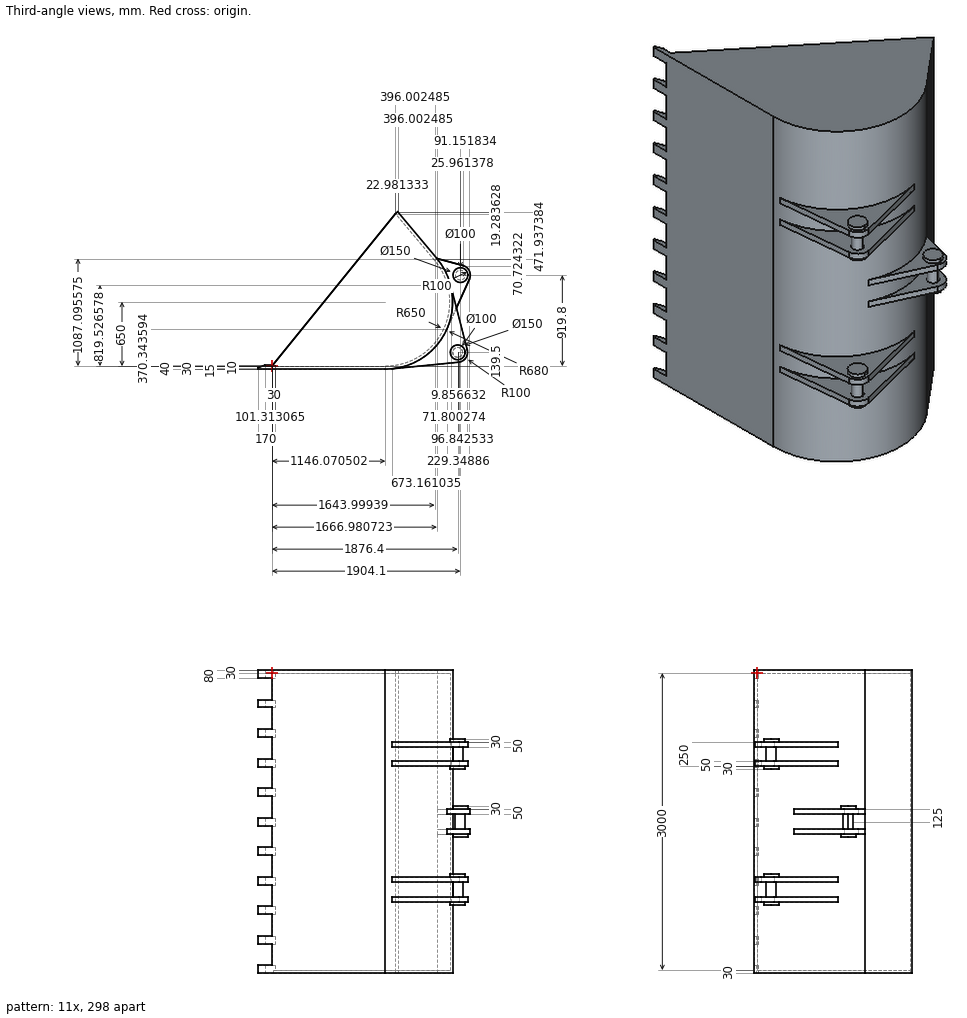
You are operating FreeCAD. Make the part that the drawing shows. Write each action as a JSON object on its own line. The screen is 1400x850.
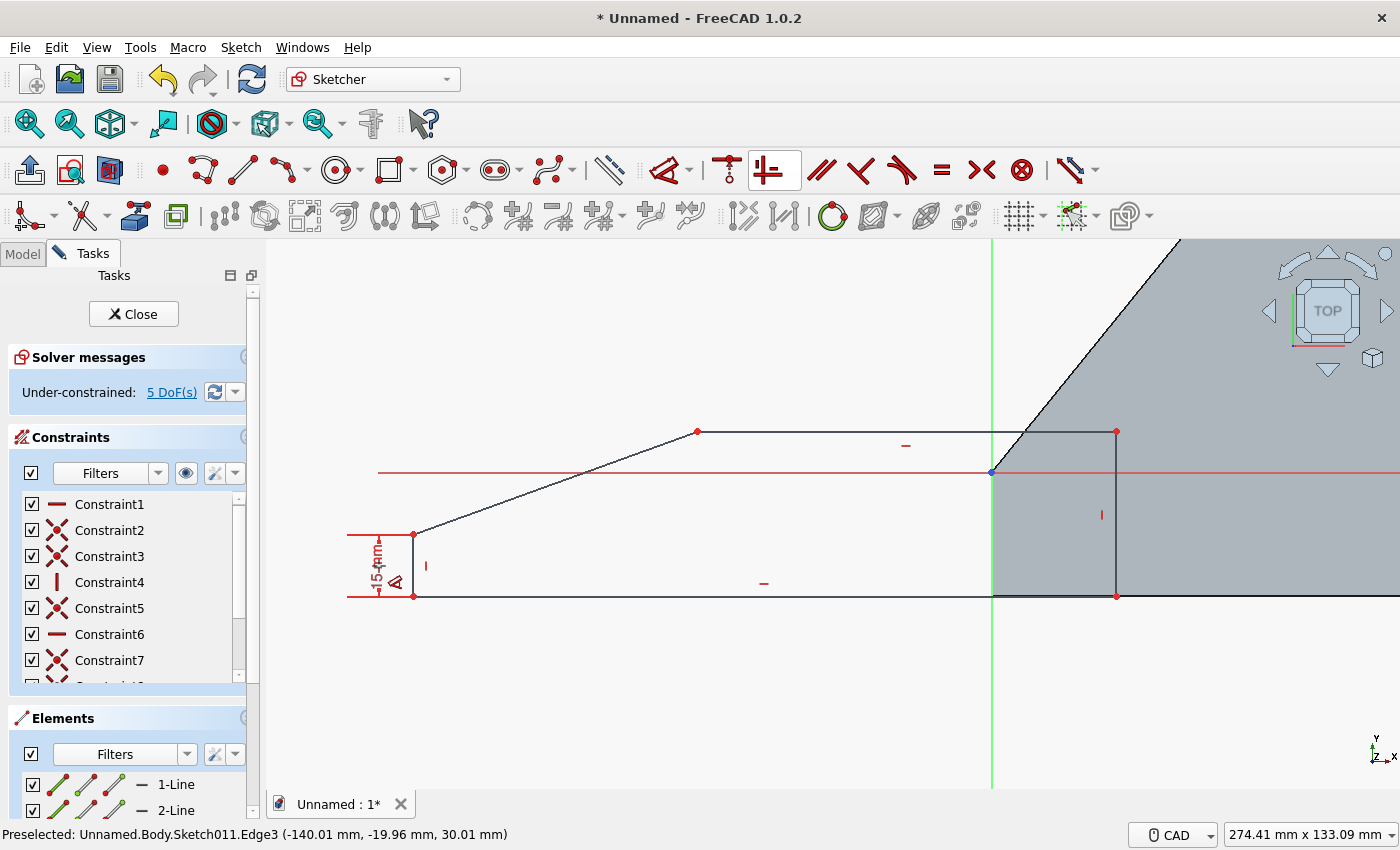
{"action": "left_click", "coordinate": [1116, 547]}
{"action": "left_click", "coordinate": [1150, 514]}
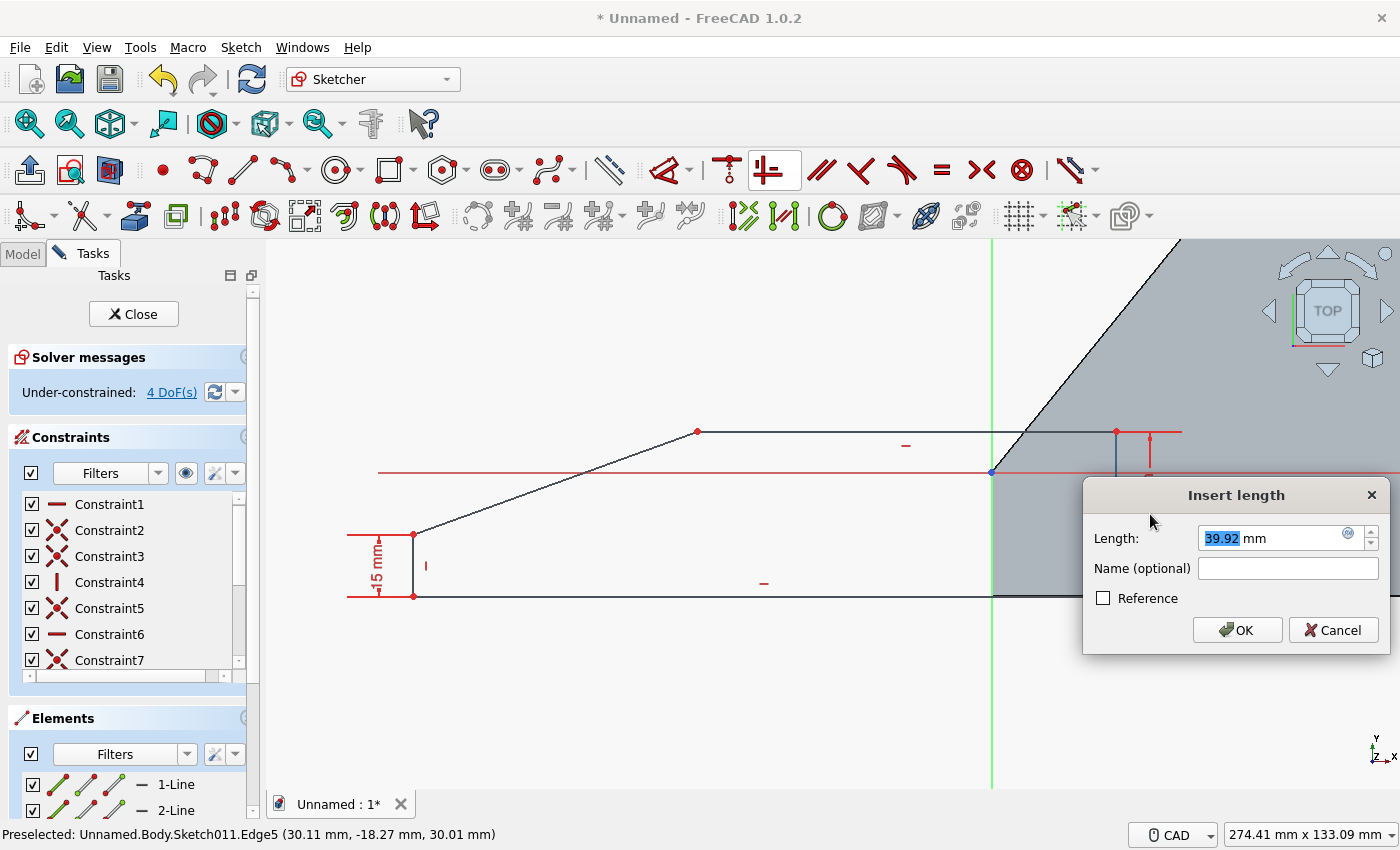
{"action": "type", "text": "40"}
{"action": "key", "text": "Return"}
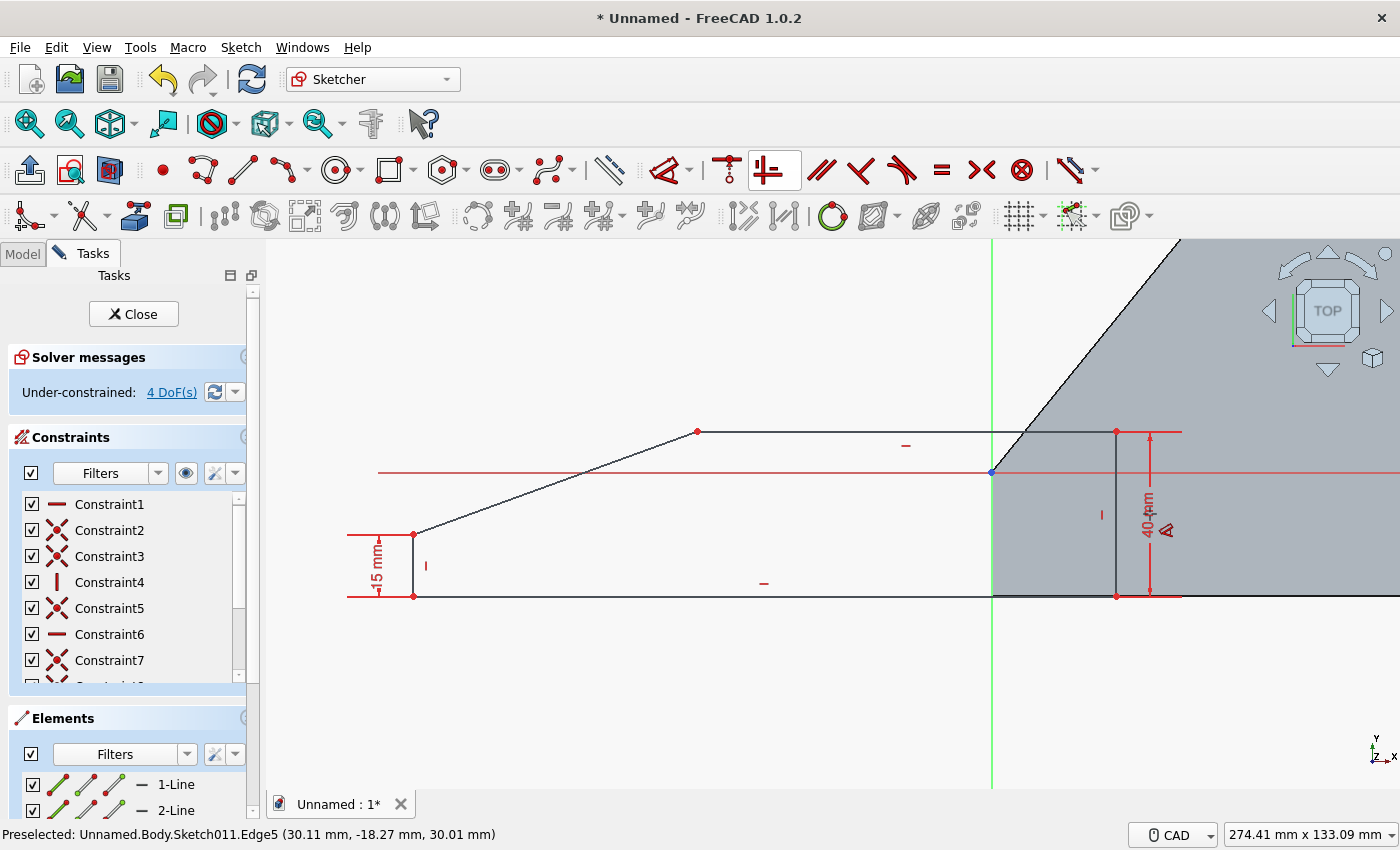
{"action": "left_click", "coordinate": [624, 597]}
{"action": "left_click", "coordinate": [764, 631]}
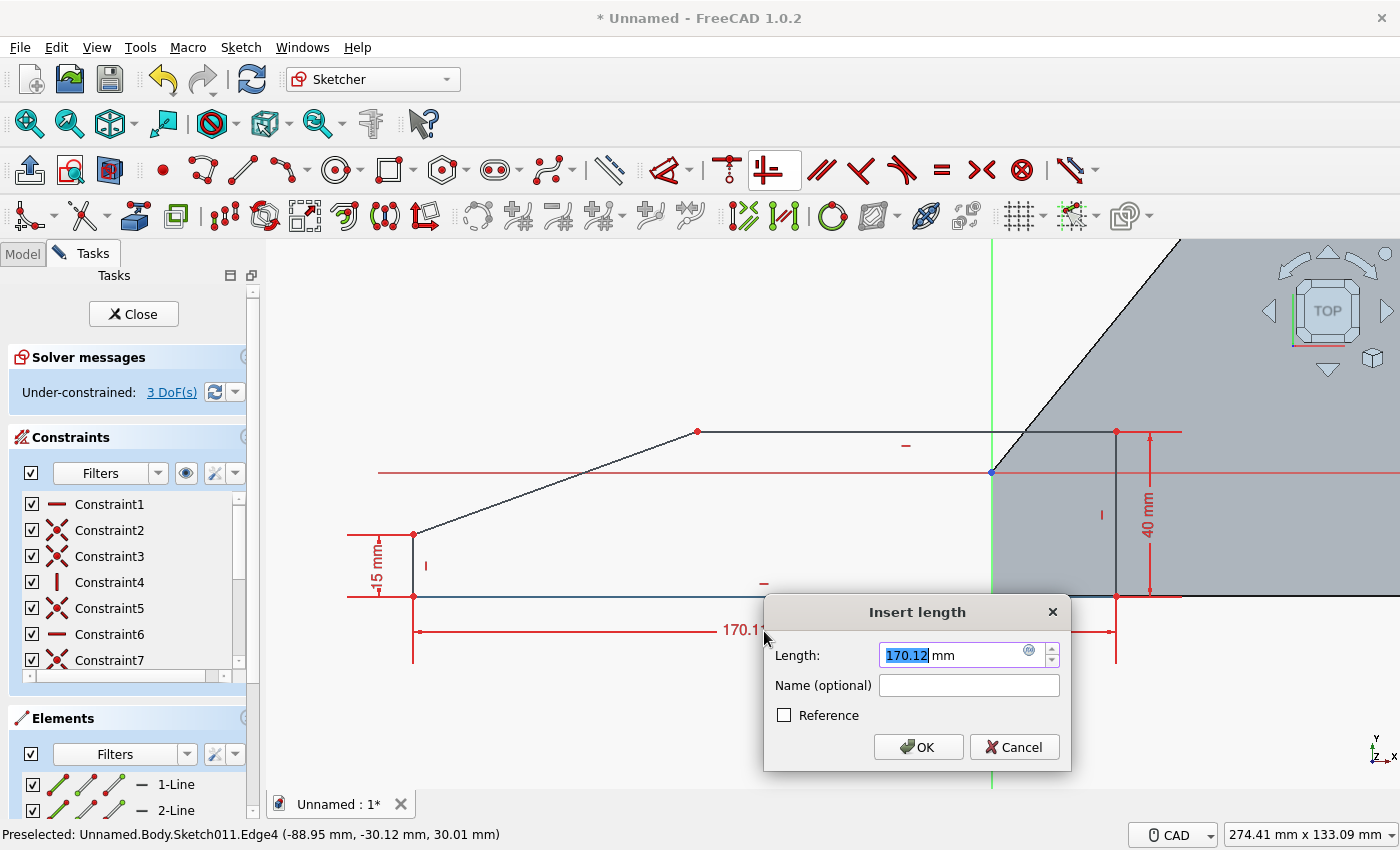
{"action": "type", "text": "170"}
{"action": "key", "text": "Return"}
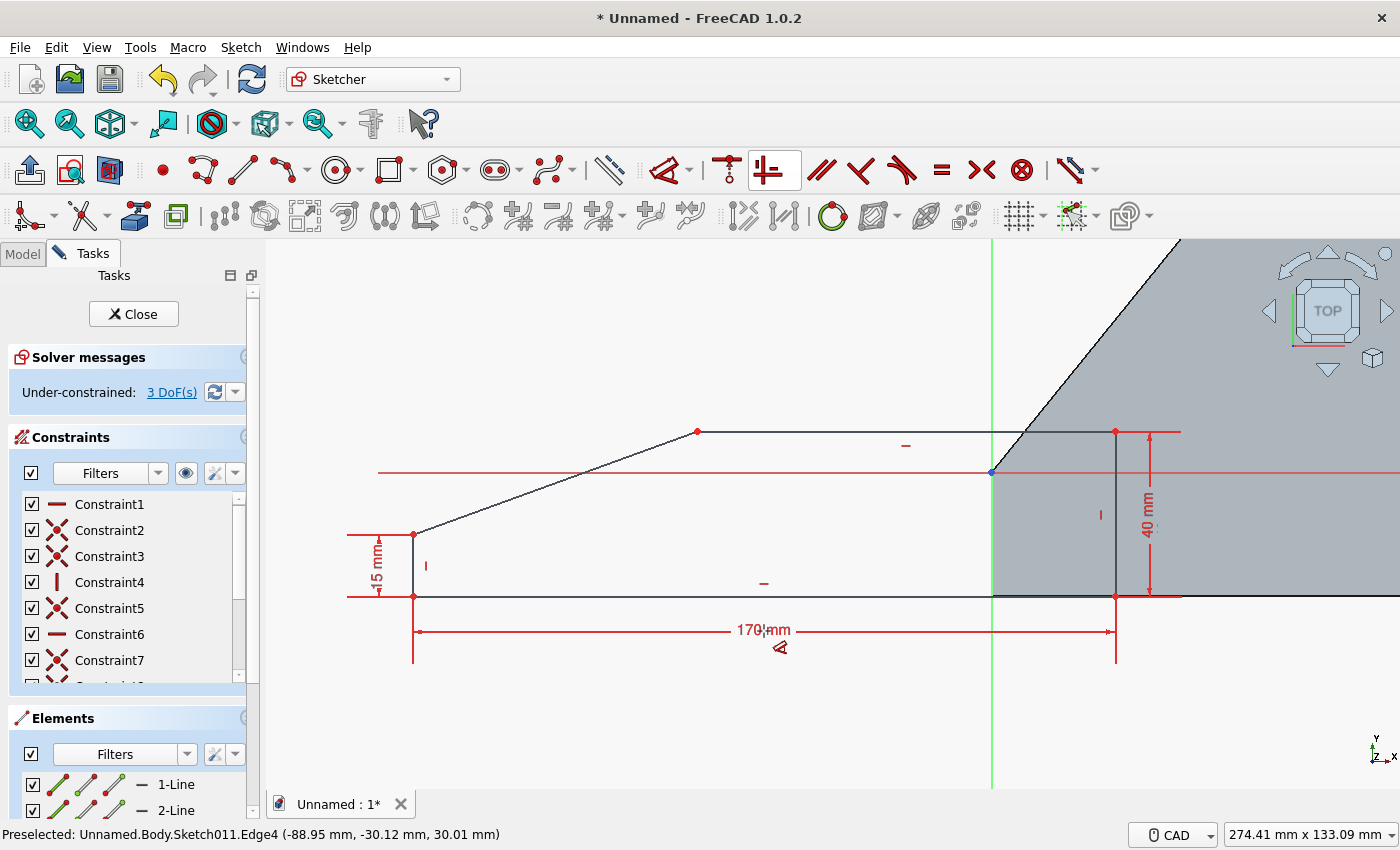
{"action": "left_click", "coordinate": [1116, 432]}
{"action": "left_click", "coordinate": [1054, 398]}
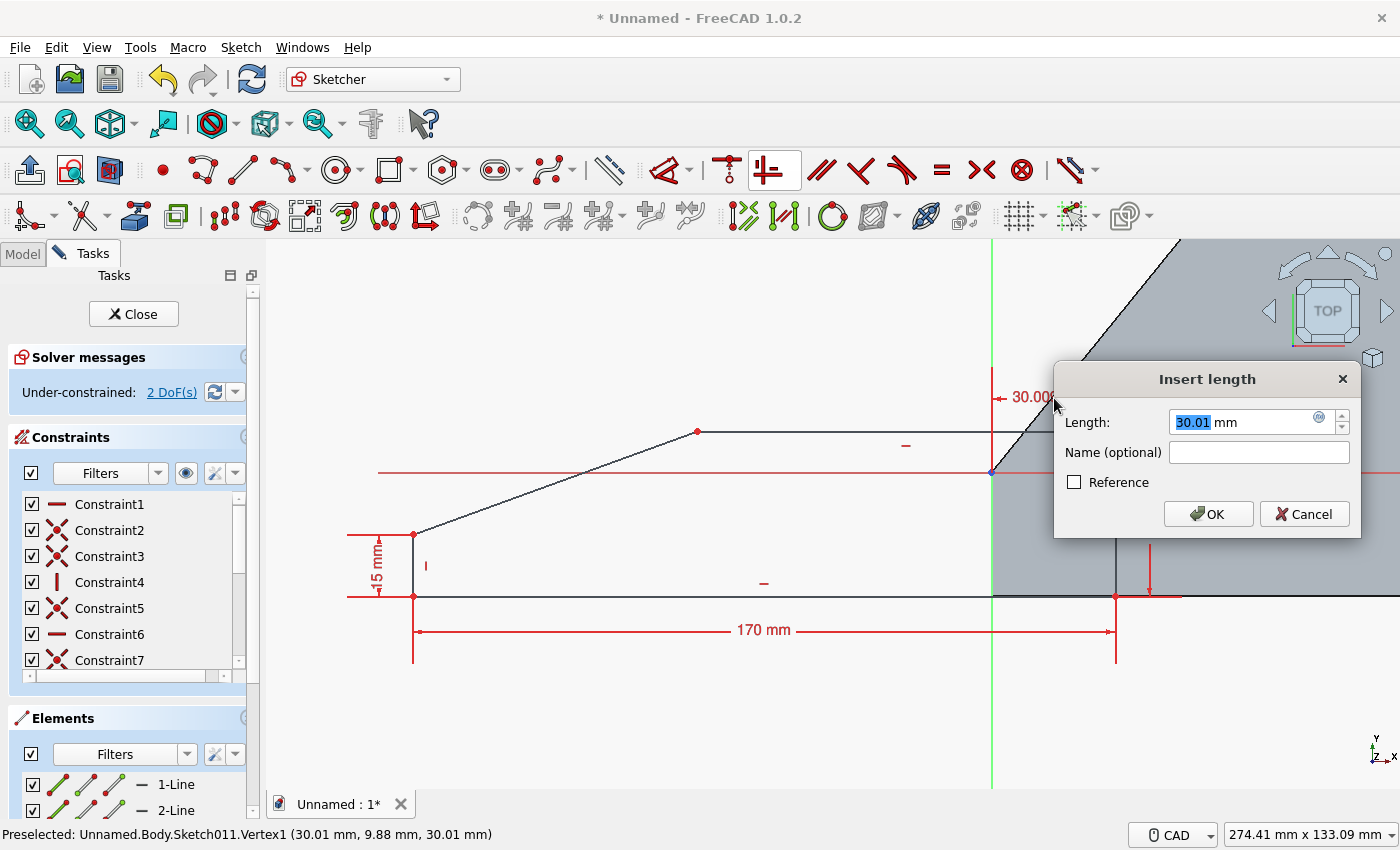
{"action": "type", "text": "30"}
{"action": "key", "text": "Return"}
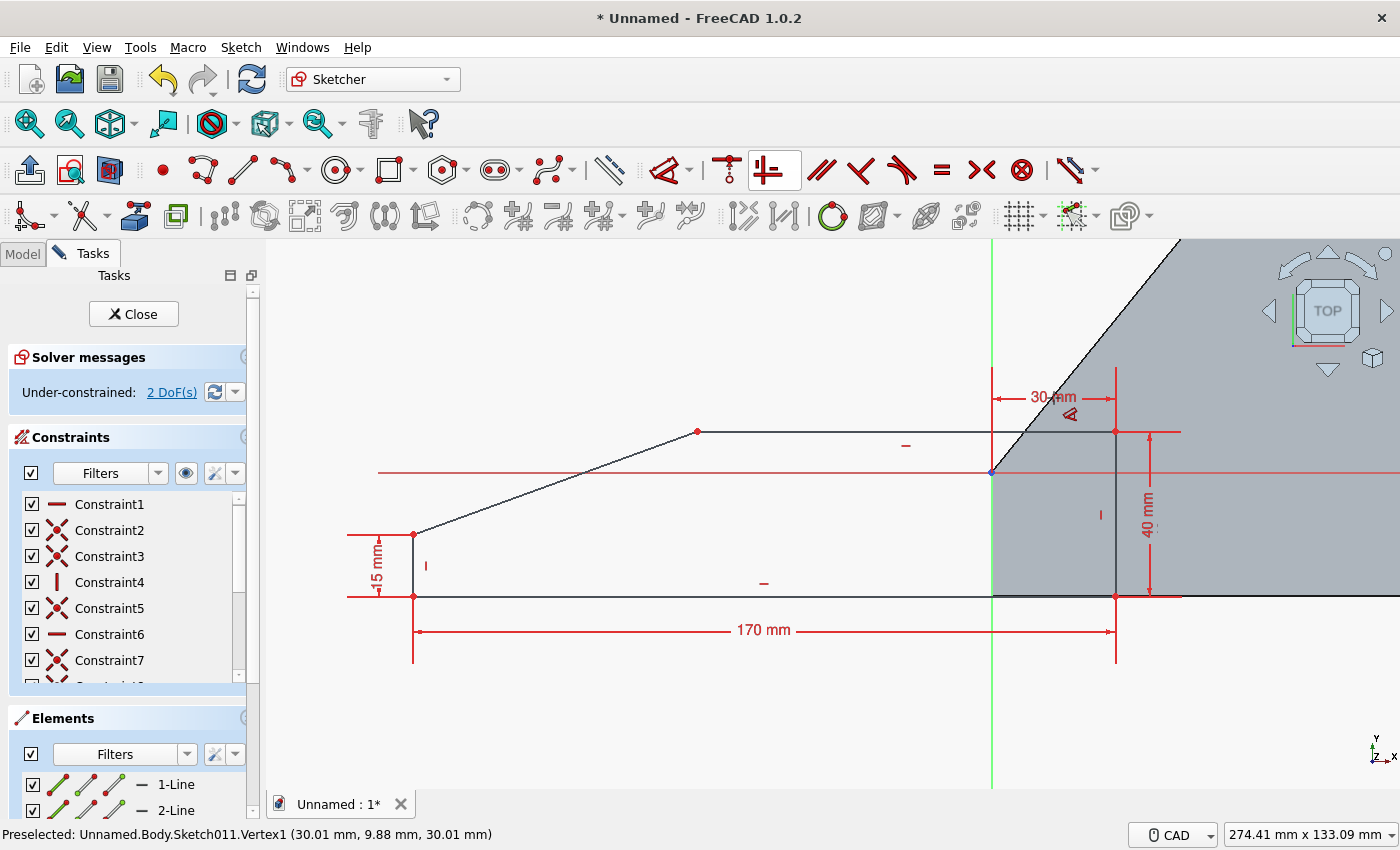
{"action": "left_click", "coordinate": [1116, 432]}
{"action": "left_click", "coordinate": [1150, 452]}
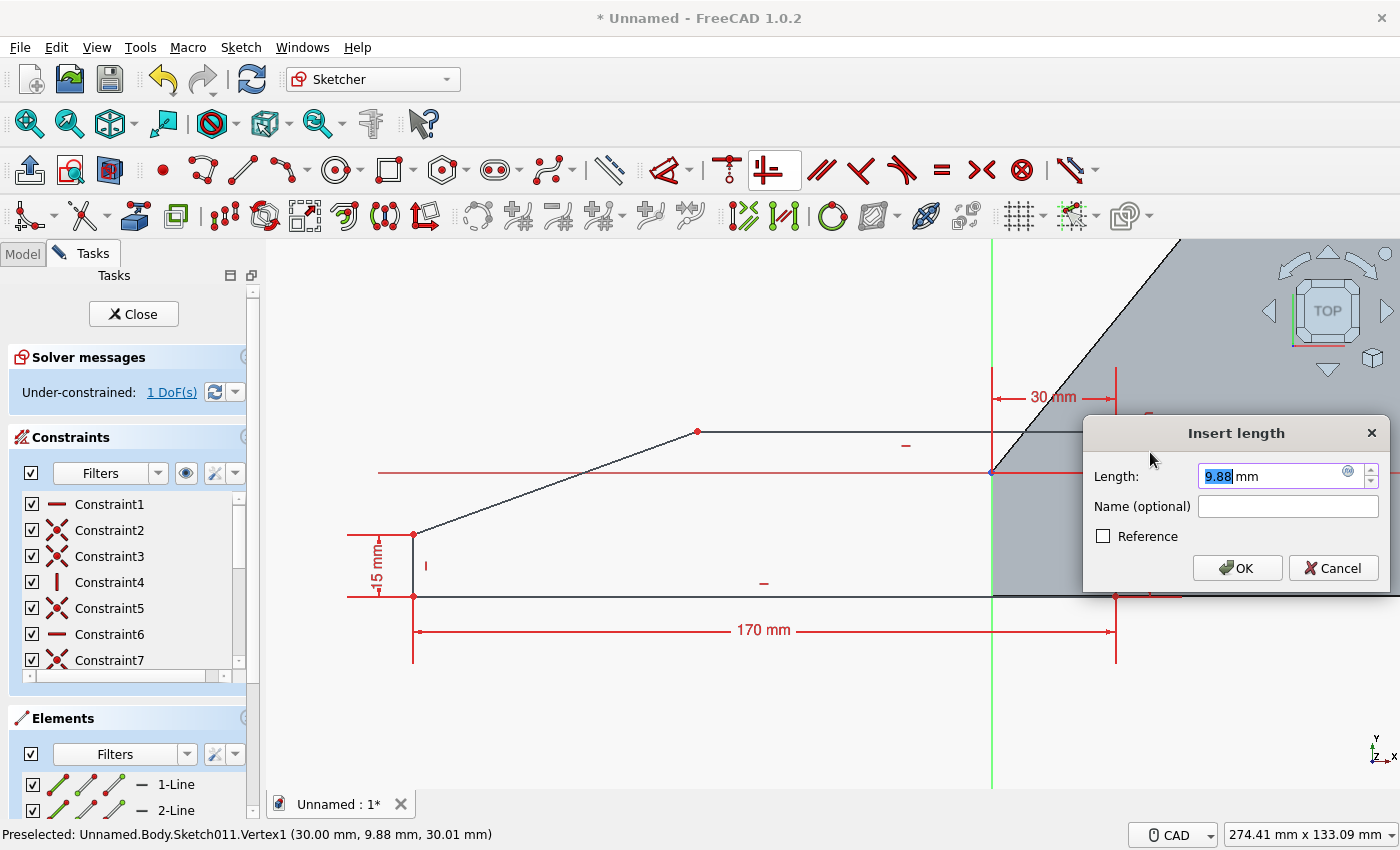
{"action": "type", "text": "10"}
{"action": "key", "text": "Return"}